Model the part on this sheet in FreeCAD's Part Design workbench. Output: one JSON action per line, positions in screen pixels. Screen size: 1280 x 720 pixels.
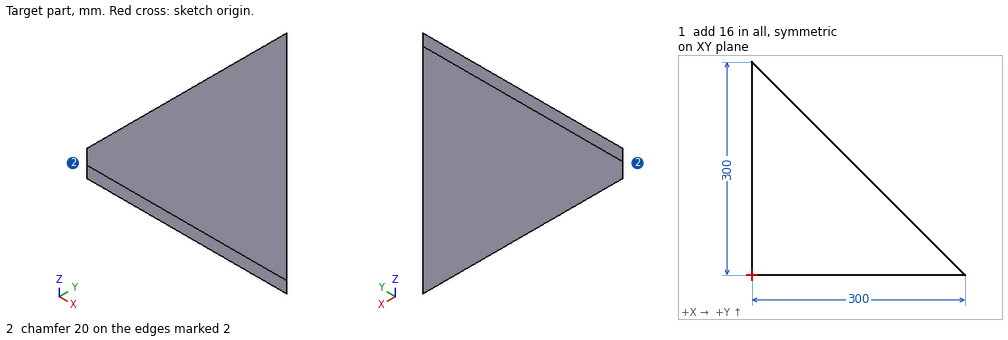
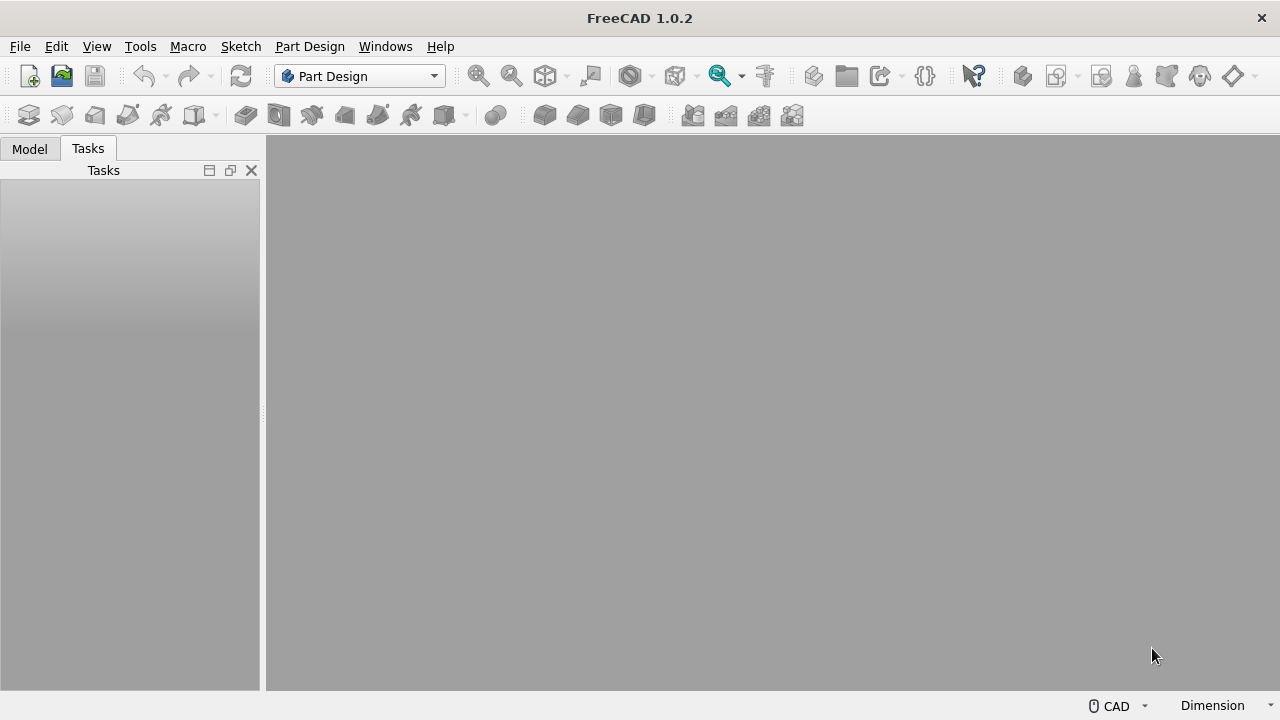
{"action": "left_click", "coordinate": [29, 76]}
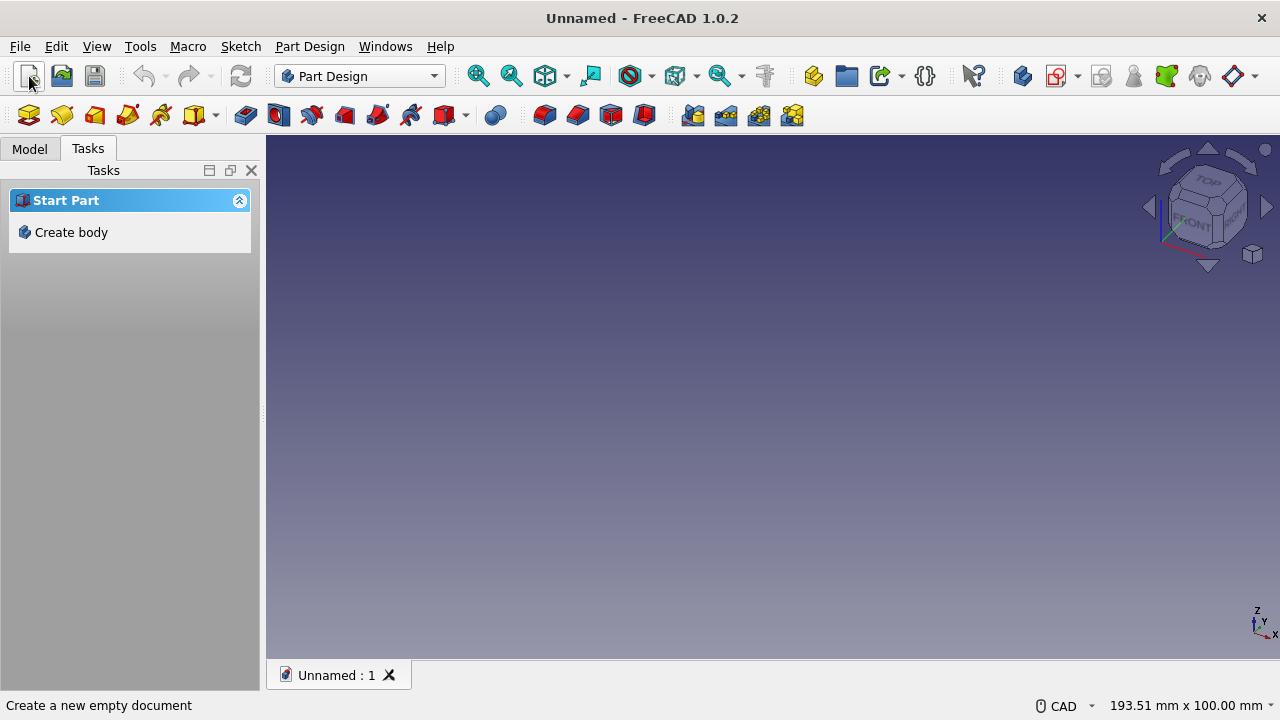
{"action": "left_click", "coordinate": [1056, 76]}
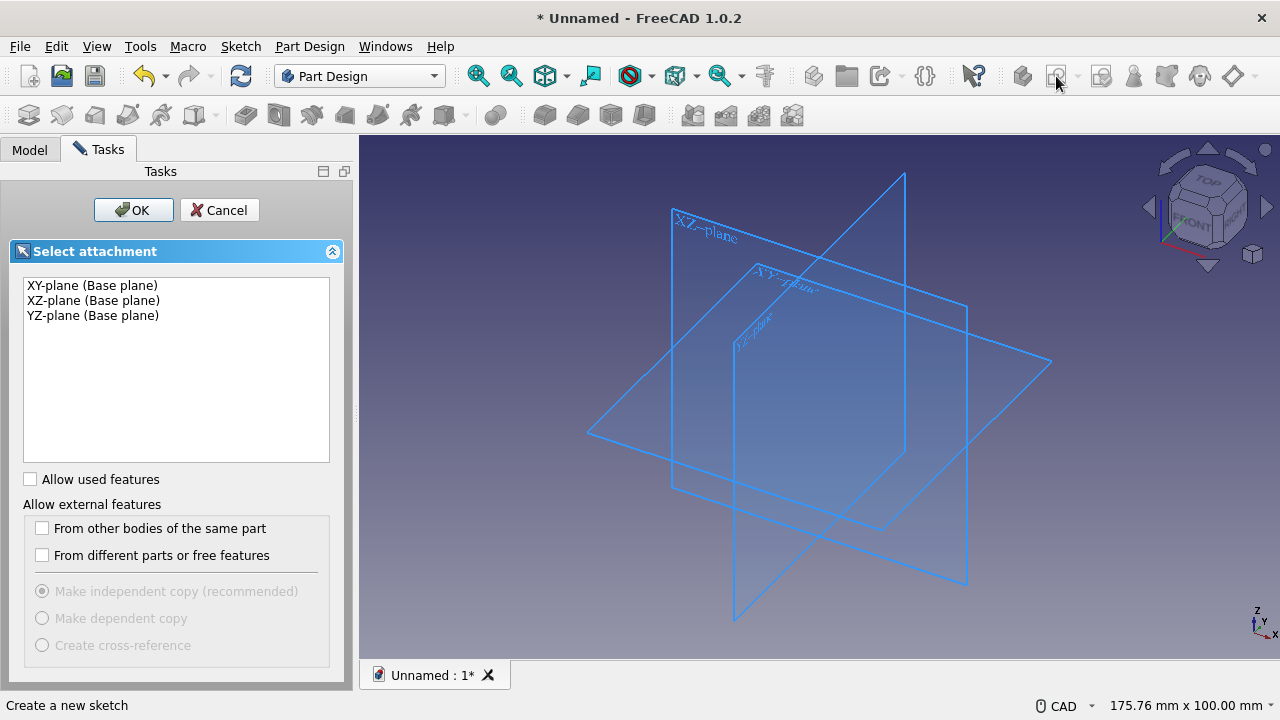
{"action": "left_click", "coordinate": [84, 286]}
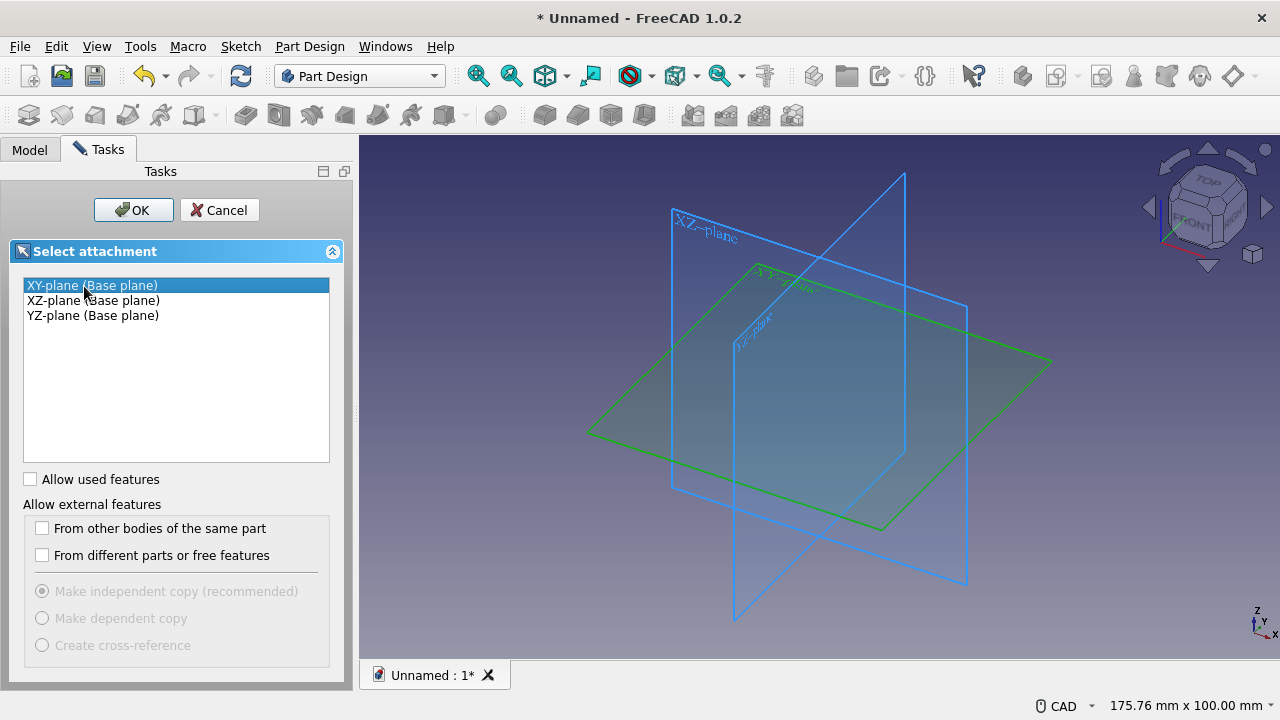
{"action": "left_click", "coordinate": [134, 210]}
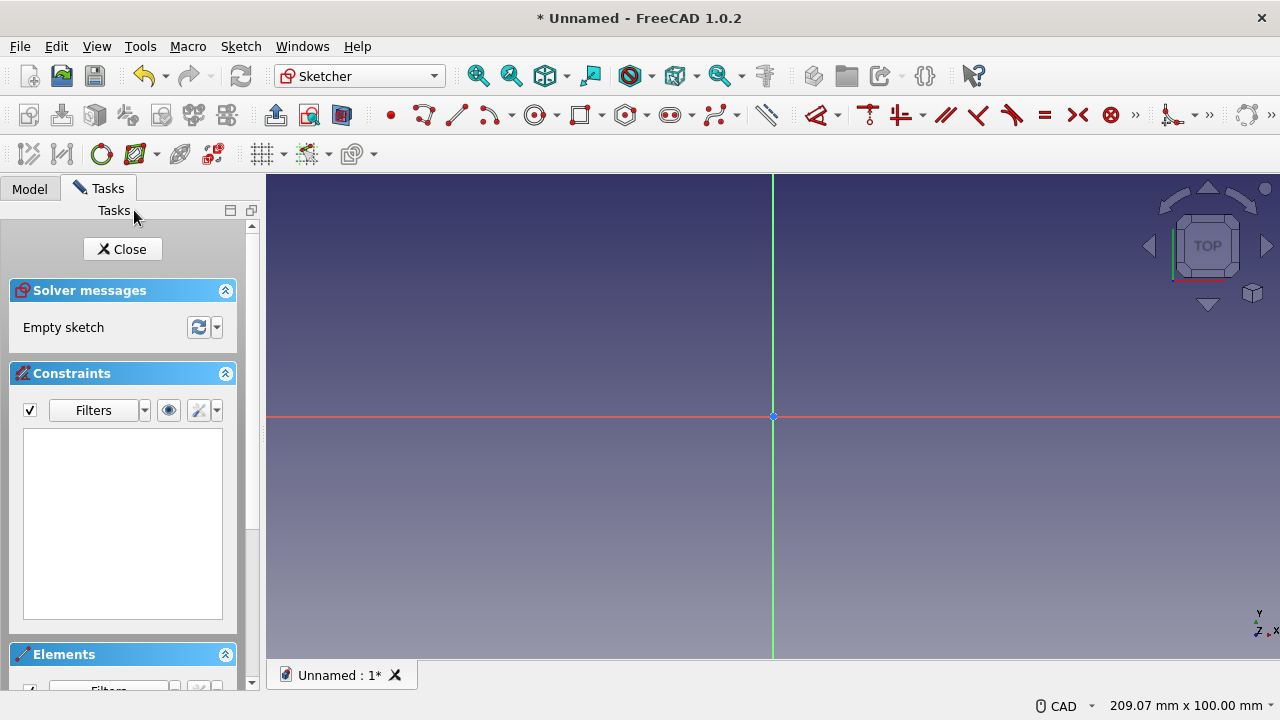
{"action": "scroll", "coordinate": [503, 601], "scroll_direction": "down", "scroll_amount": 8}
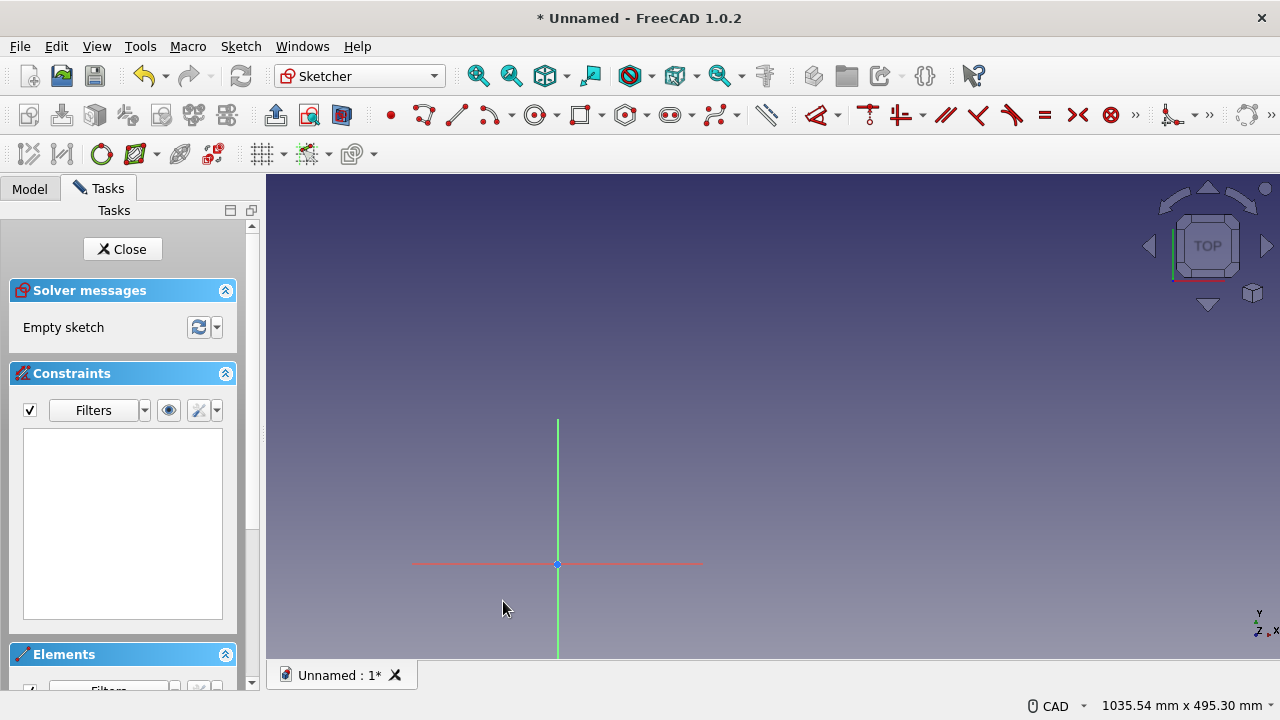
{"action": "left_click", "coordinate": [424, 116]}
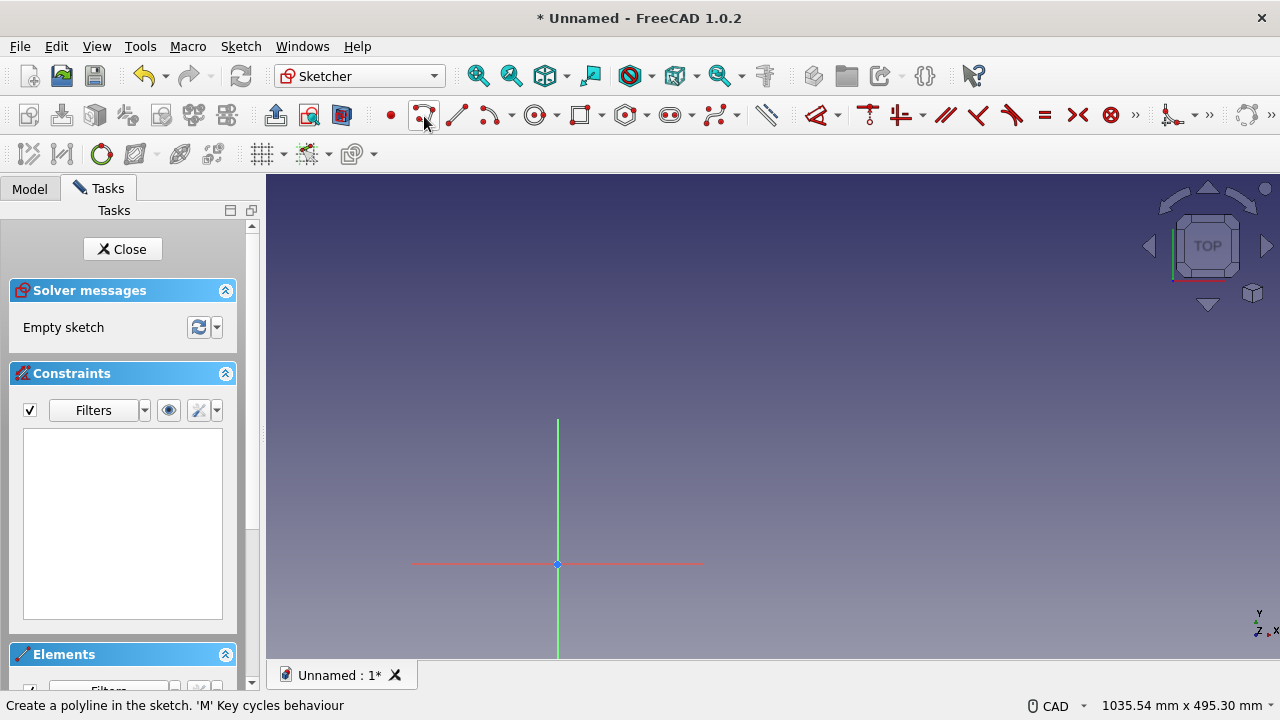
{"action": "left_click", "coordinate": [558, 564]}
{"action": "left_click", "coordinate": [851, 555]}
{"action": "left_click", "coordinate": [567, 271]}
{"action": "left_click", "coordinate": [558, 564]}
{"action": "key", "text": "Escape"}
{"action": "key", "text": "Escape"}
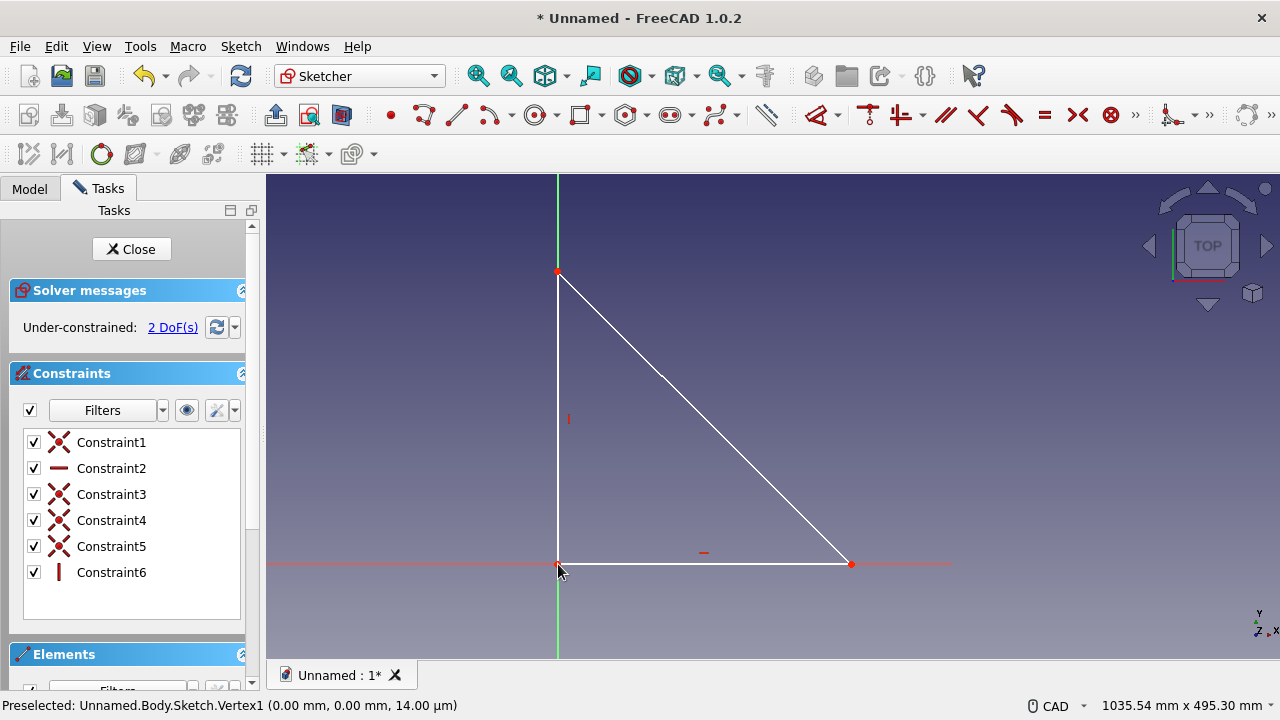
{"action": "left_click", "coordinate": [646, 564]}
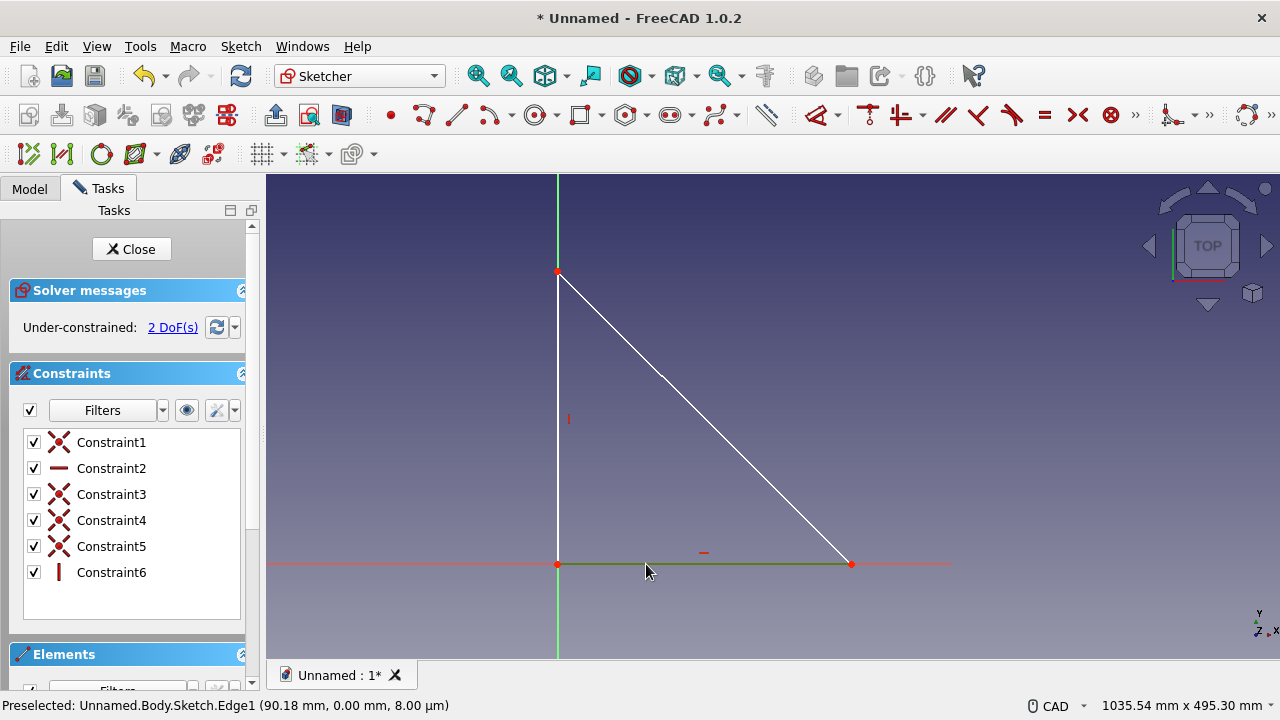
{"action": "key", "text": "l"}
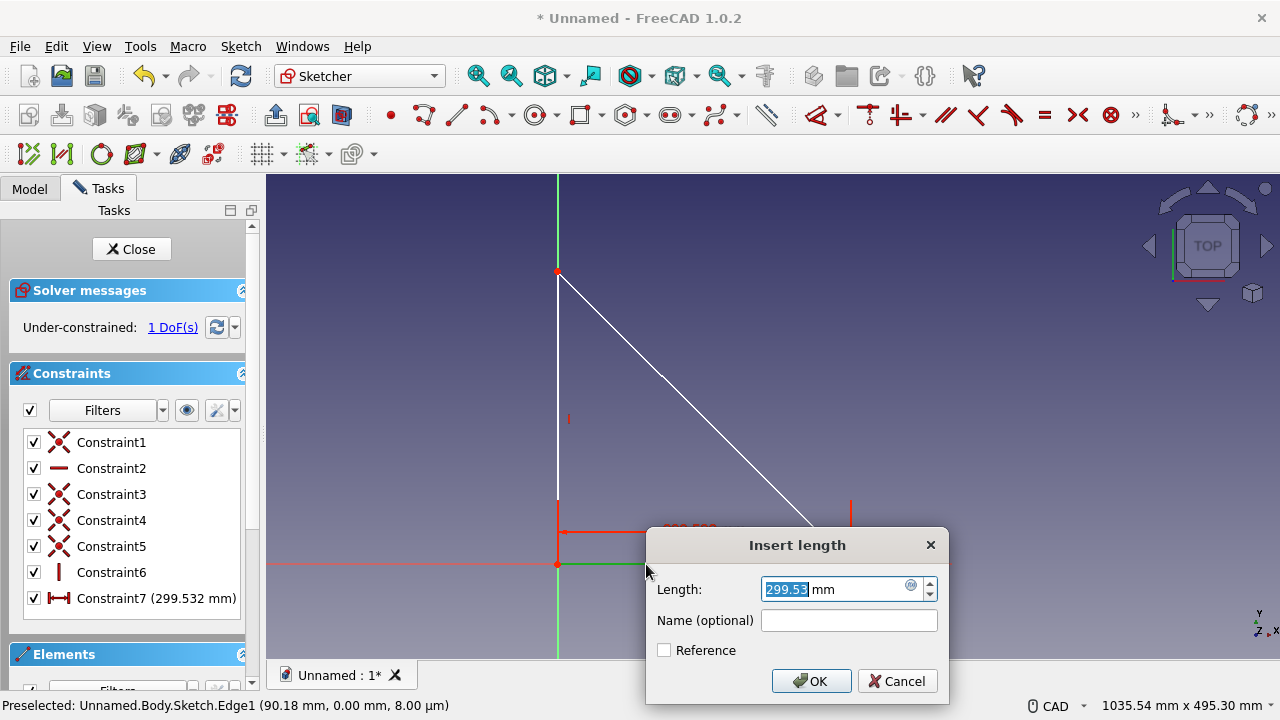
{"action": "type", "text": "300"}
{"action": "key", "text": "Return"}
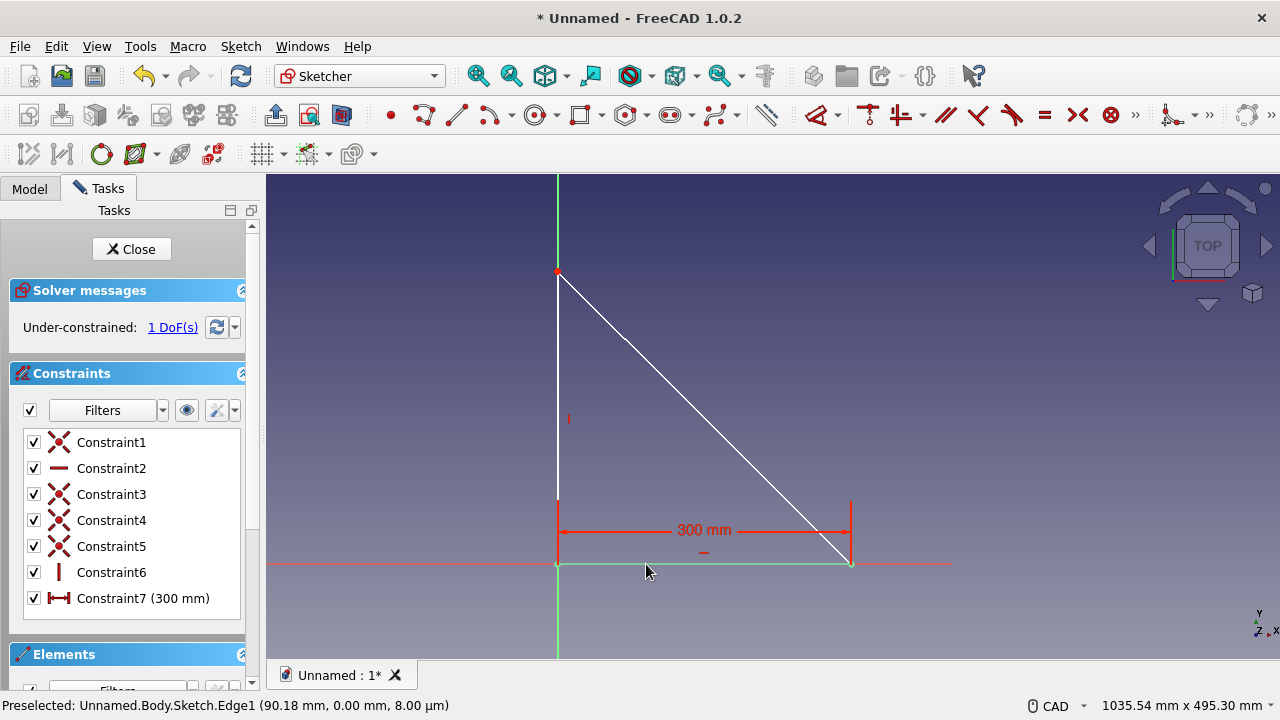
{"action": "left_click", "coordinate": [558, 360]}